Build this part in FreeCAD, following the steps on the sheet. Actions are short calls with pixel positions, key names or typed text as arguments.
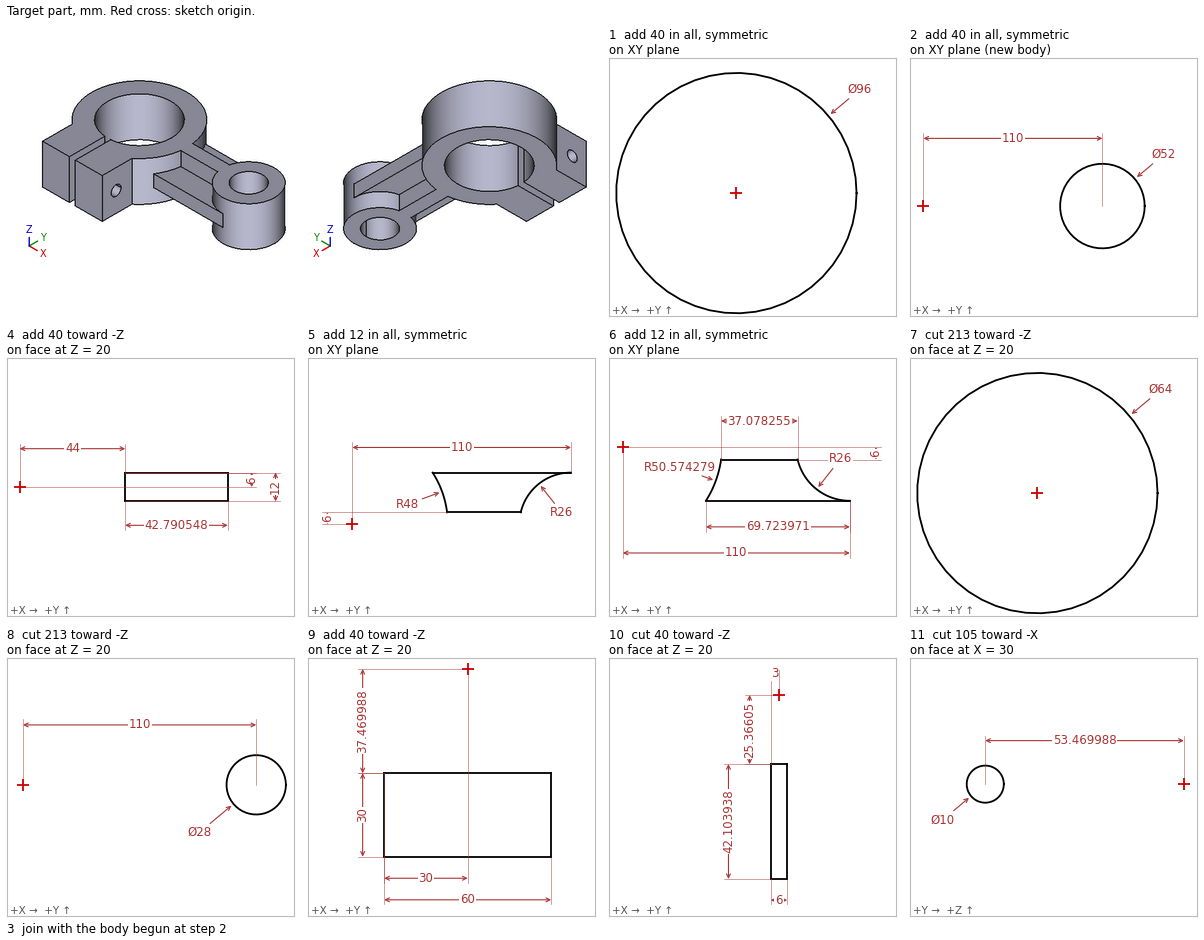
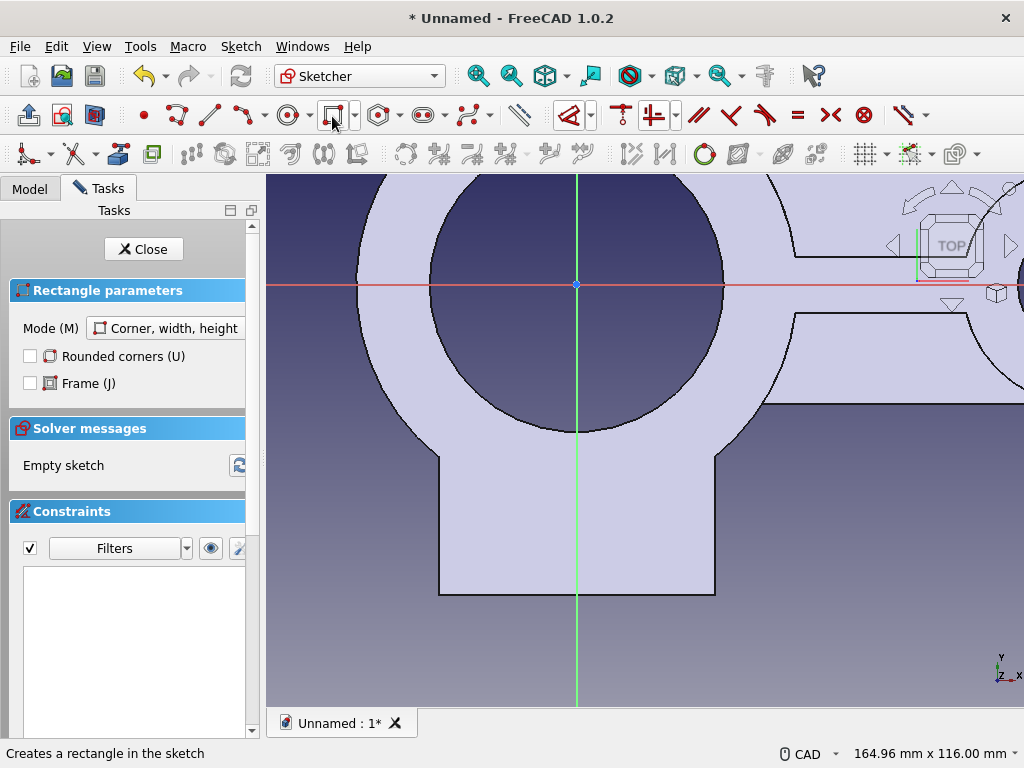
click(563, 402)
click(590, 595)
key(Escape)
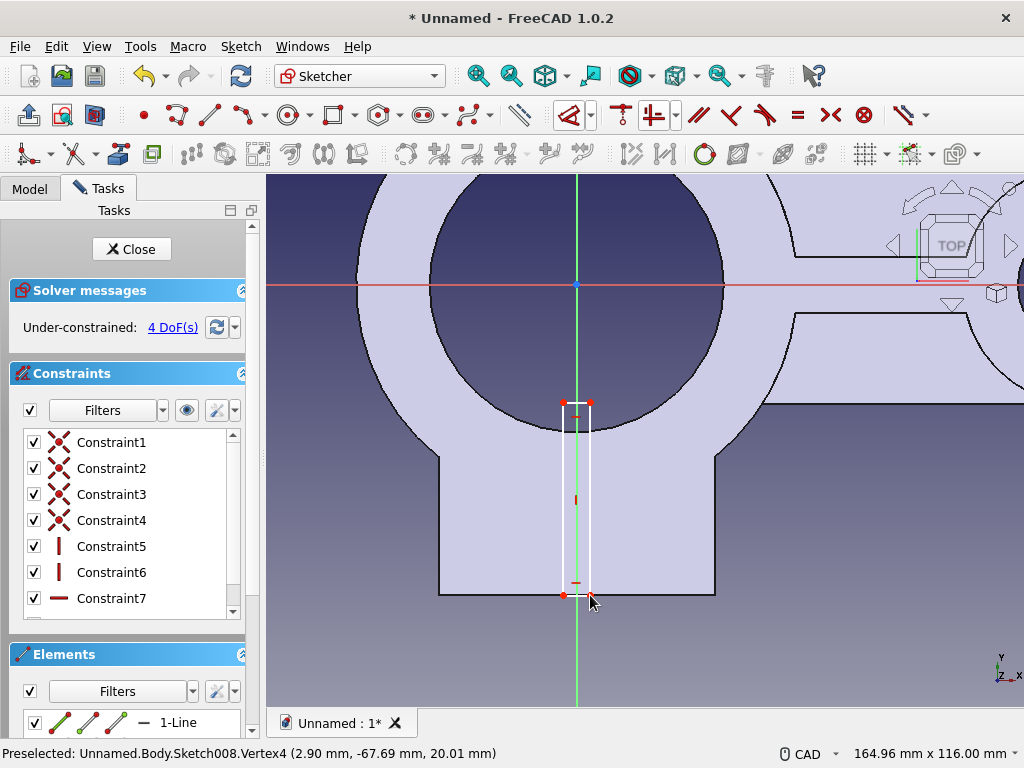
scroll(574, 596, up, 2)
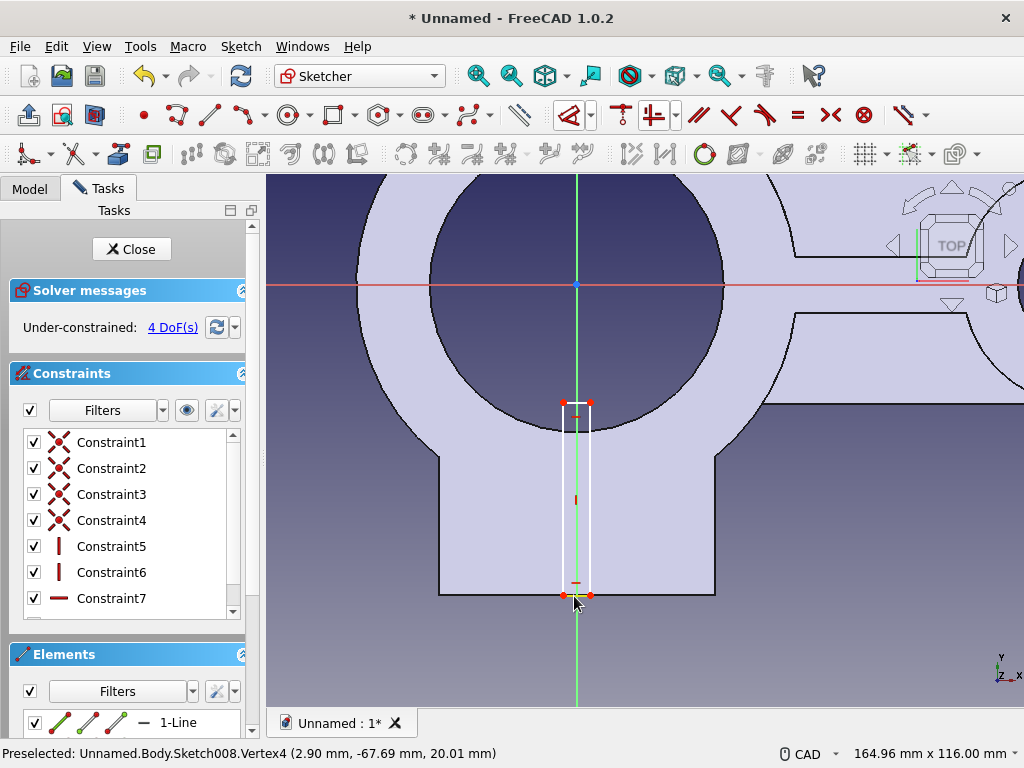
click(574, 596)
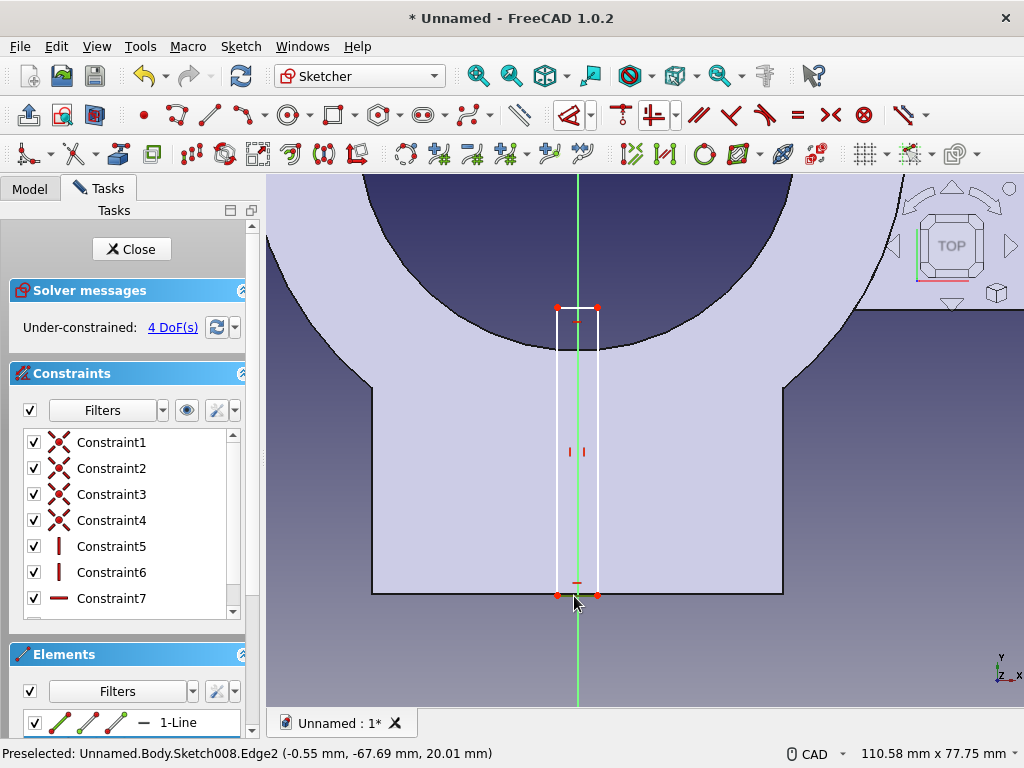
click(590, 116)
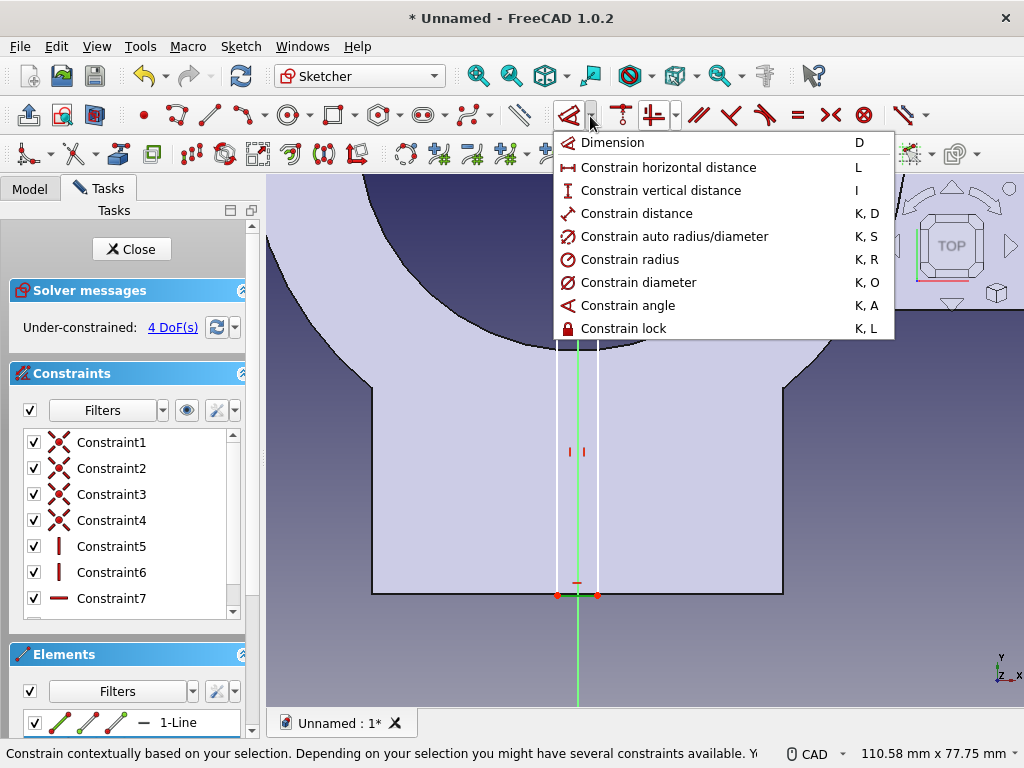
click(724, 168)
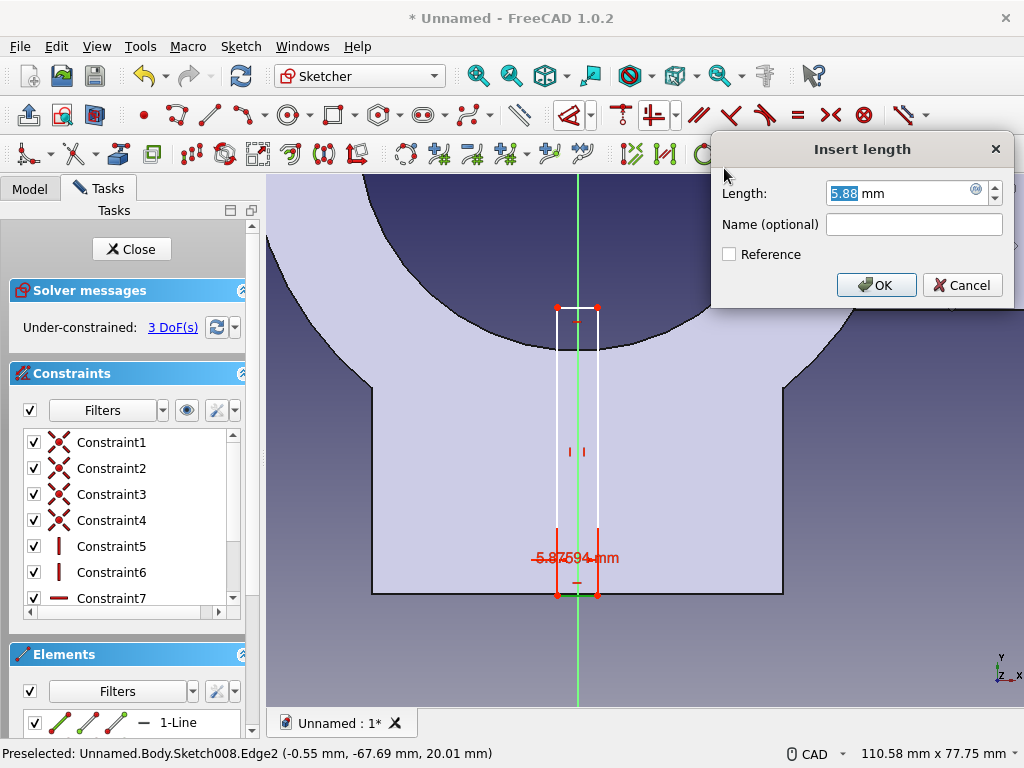
text(6)
key(Return)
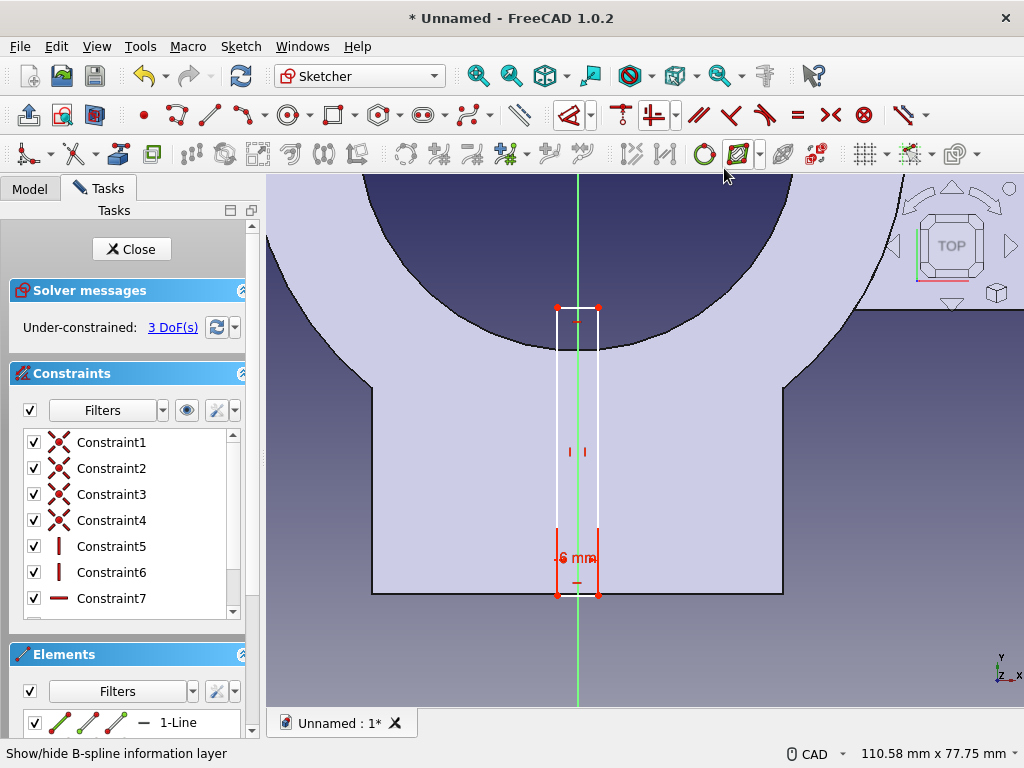
scroll(557, 308, up, 4)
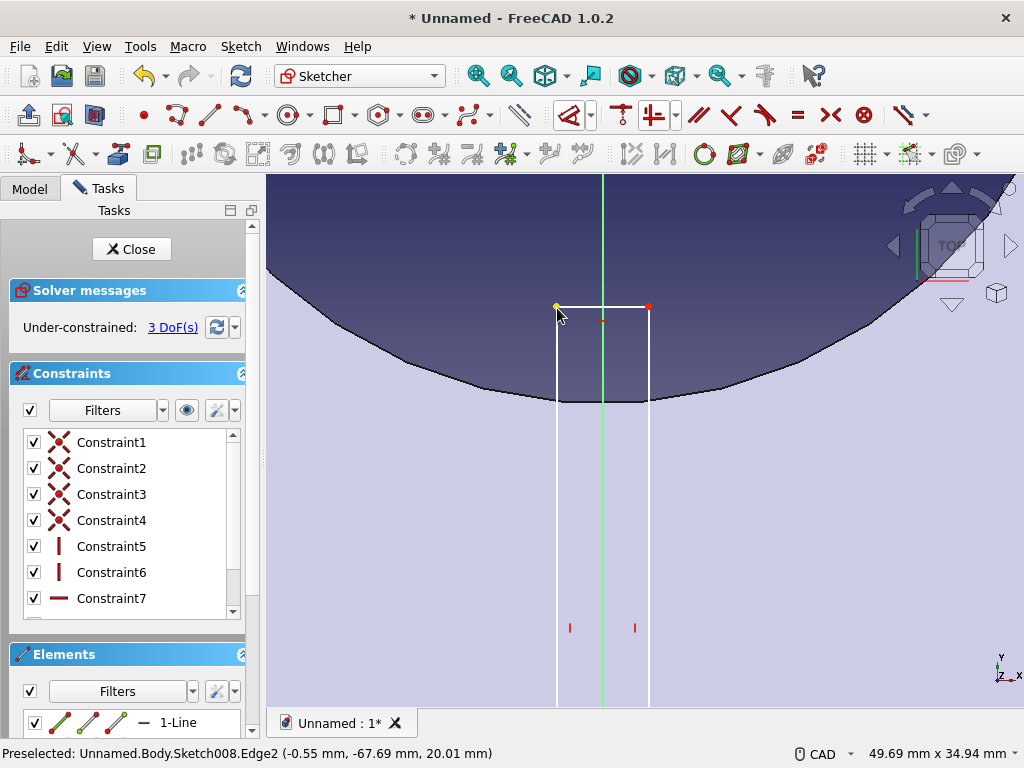
click(557, 307)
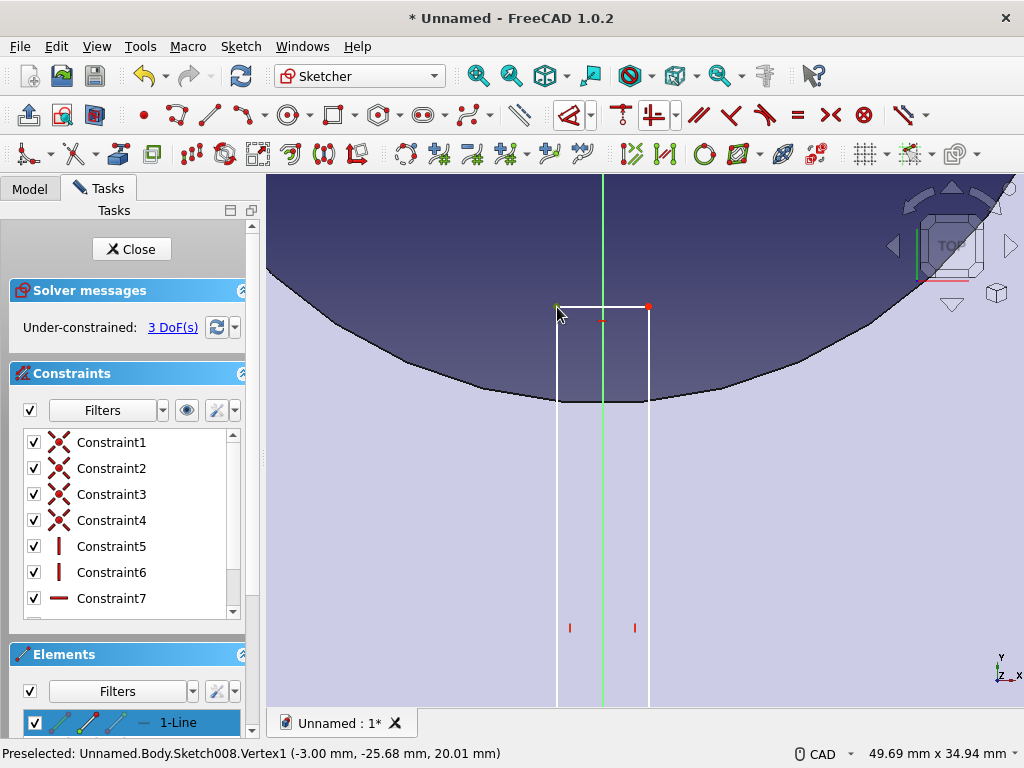
click(590, 116)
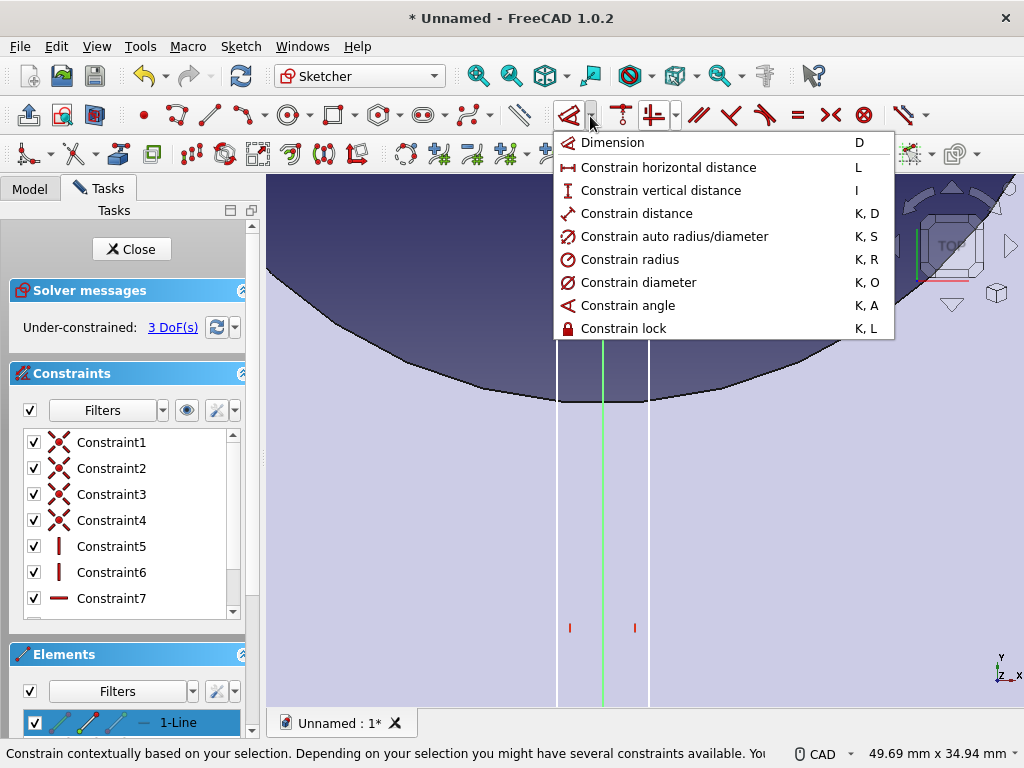
click(724, 168)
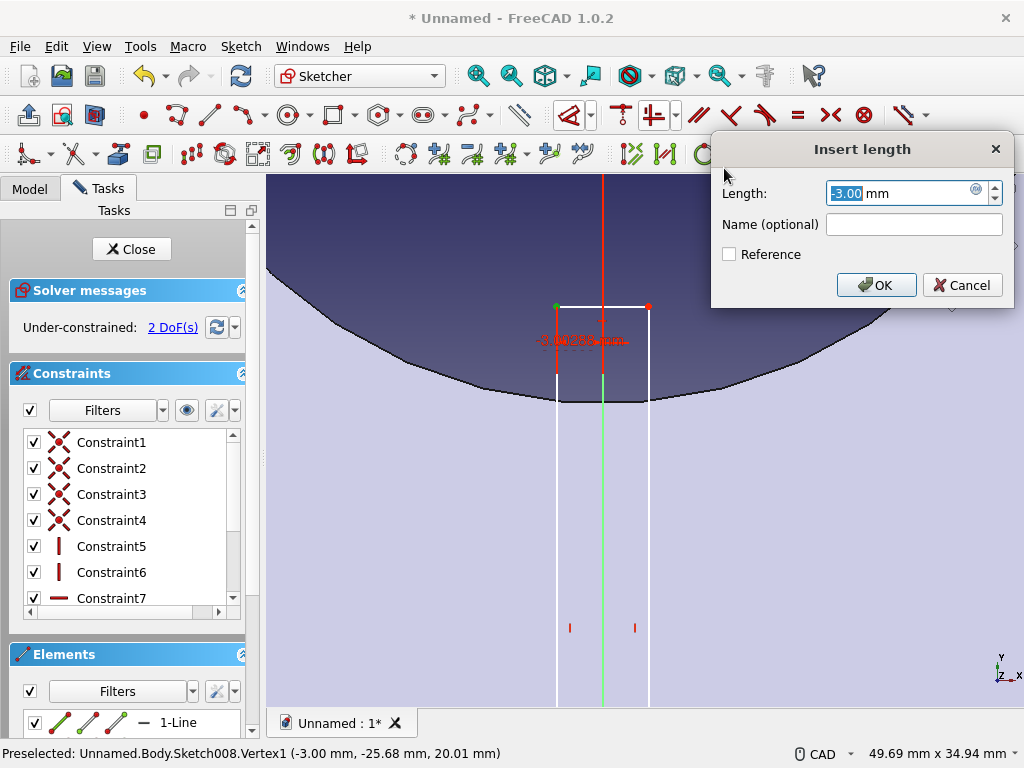
text(-3)
key(Return)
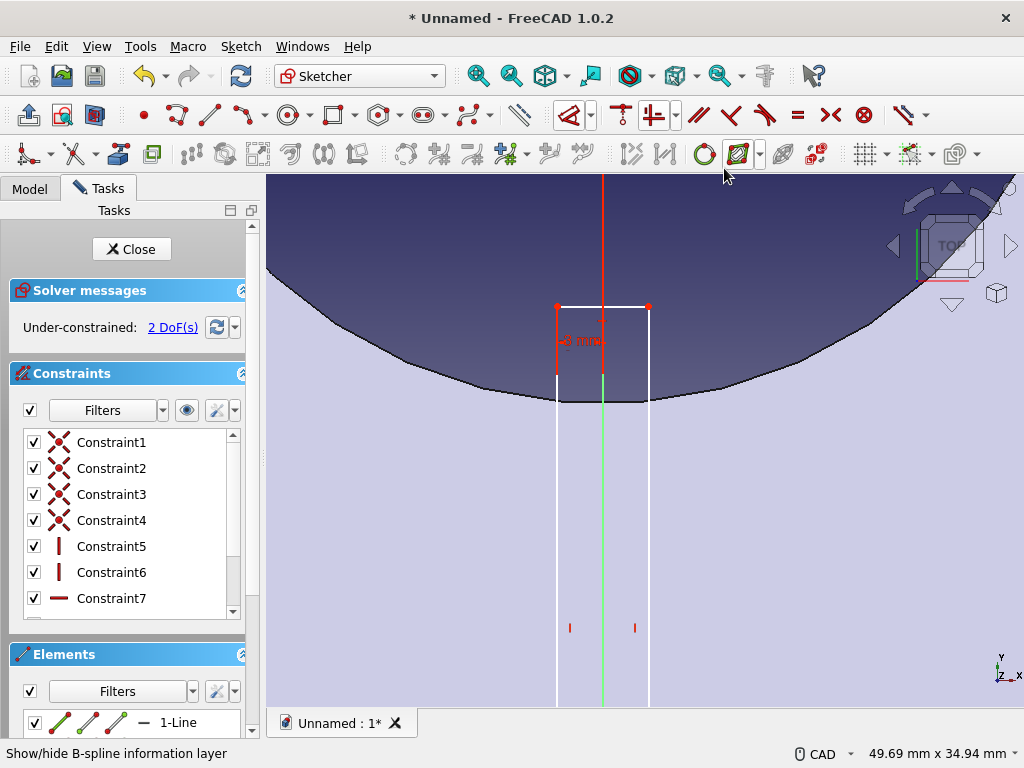
click(557, 499)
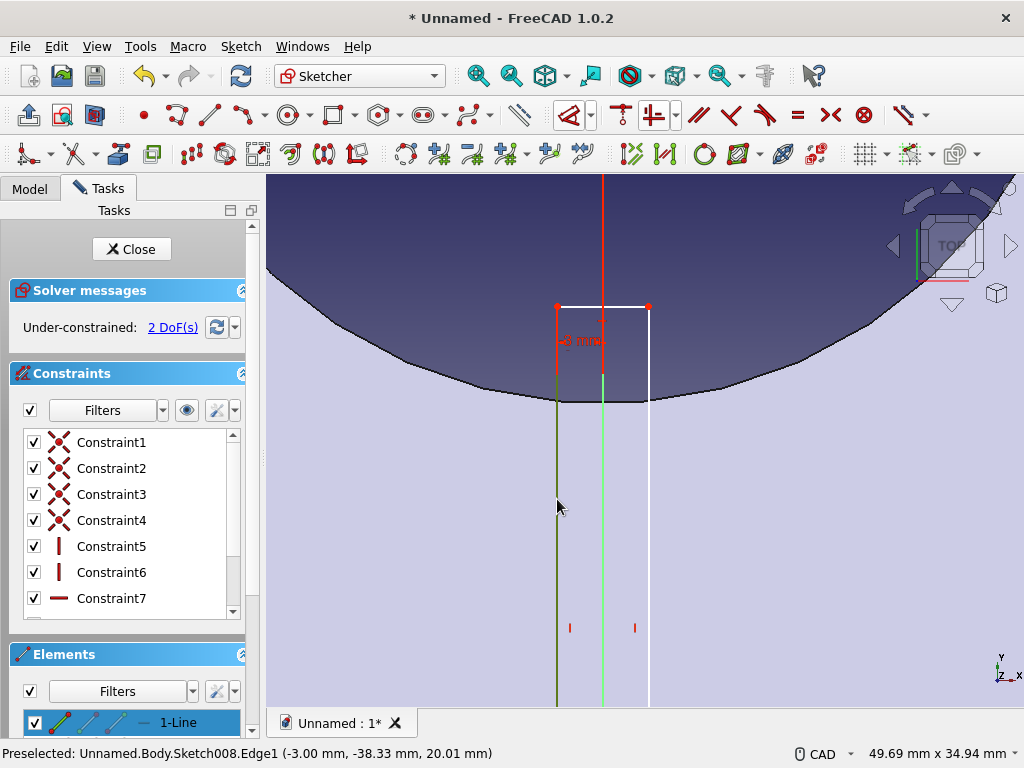
key(i)